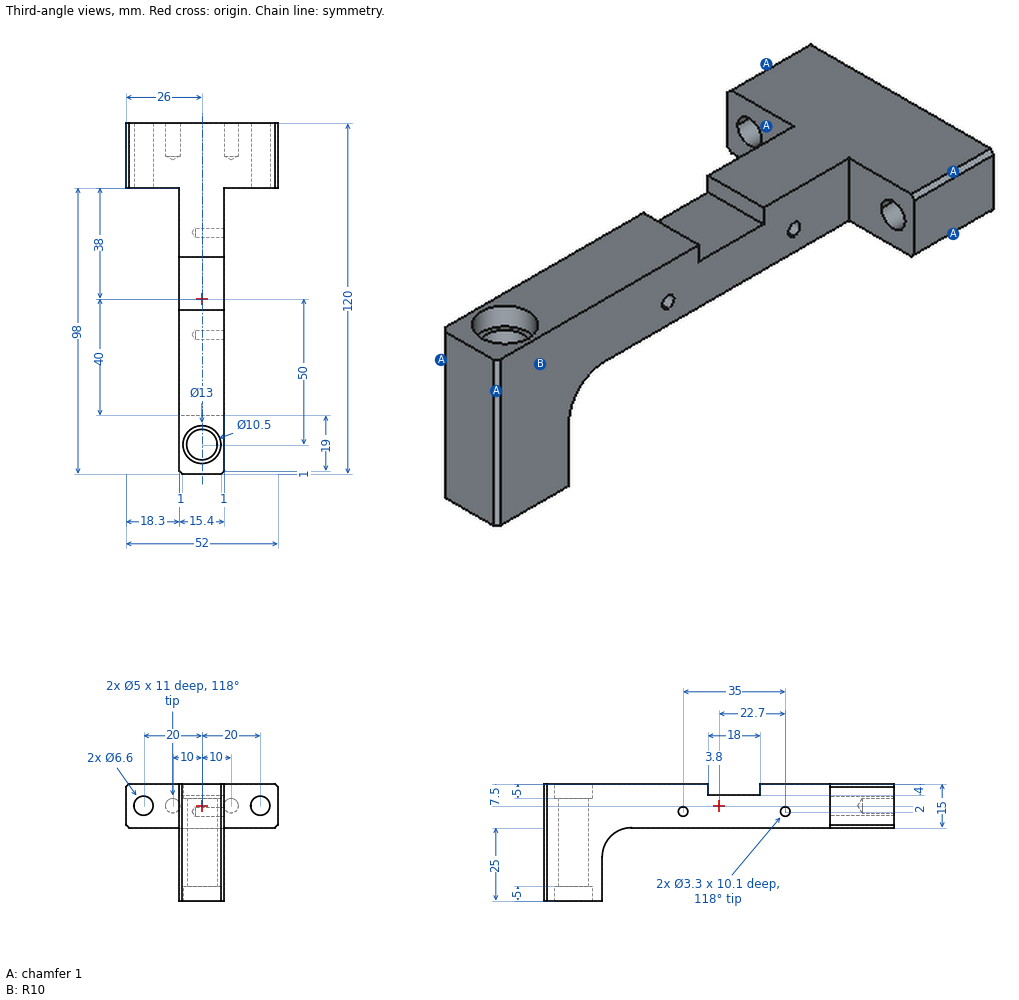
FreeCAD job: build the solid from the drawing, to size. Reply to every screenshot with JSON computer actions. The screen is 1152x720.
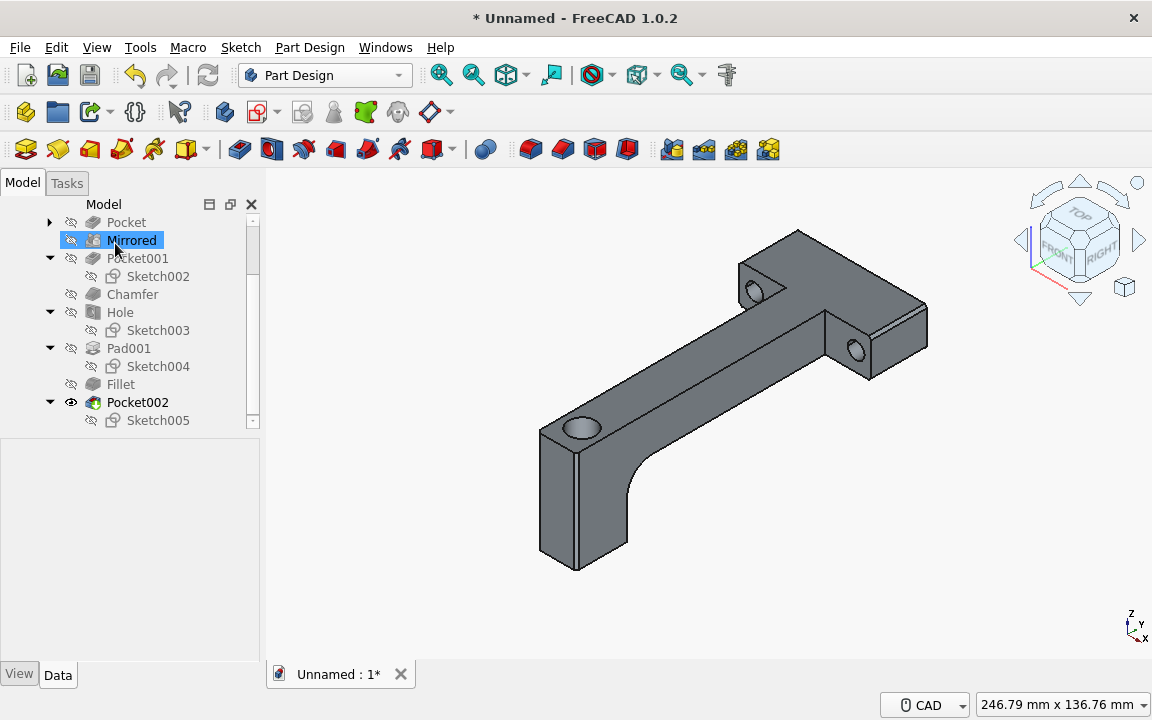
{"action": "left_click", "coordinate": [876, 299]}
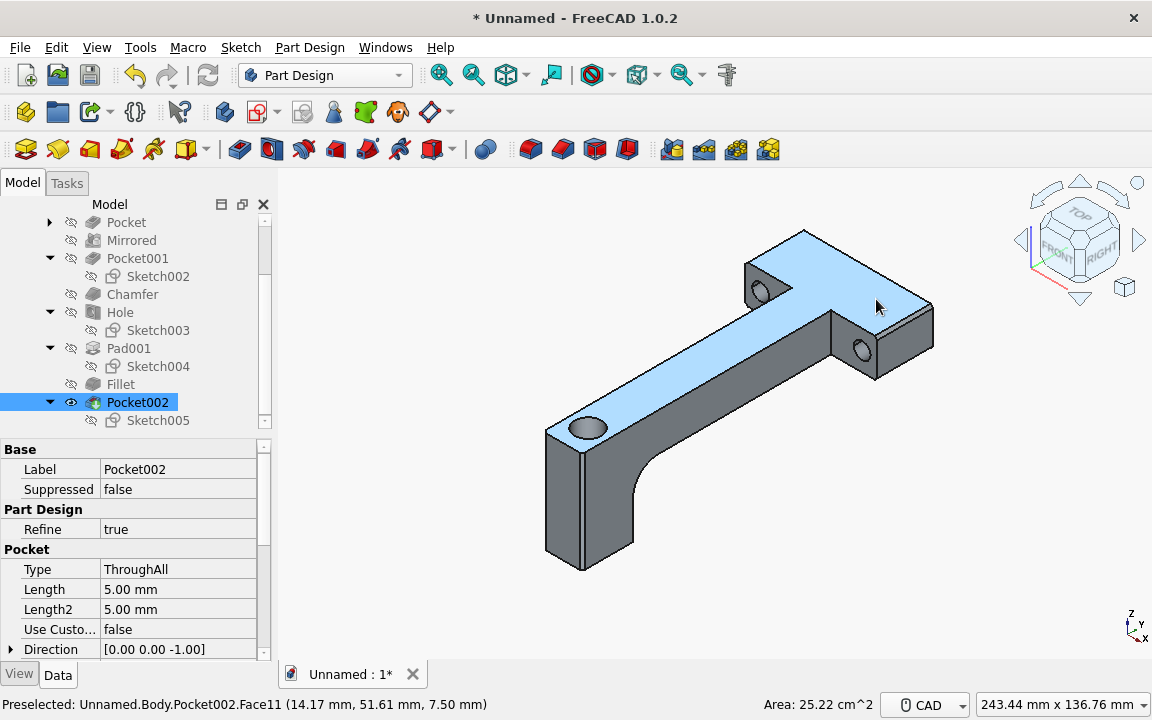
{"action": "left_click", "coordinate": [258, 112]}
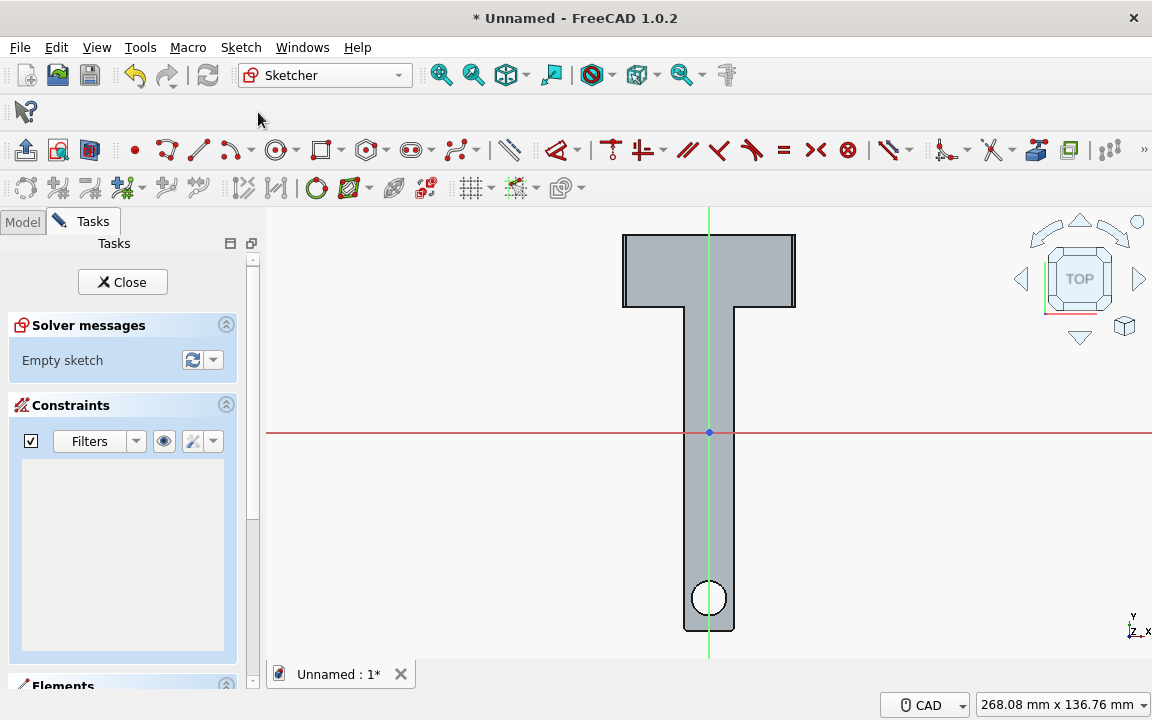
{"action": "scroll", "coordinate": [723, 631], "scroll_direction": "up", "scroll_amount": 9}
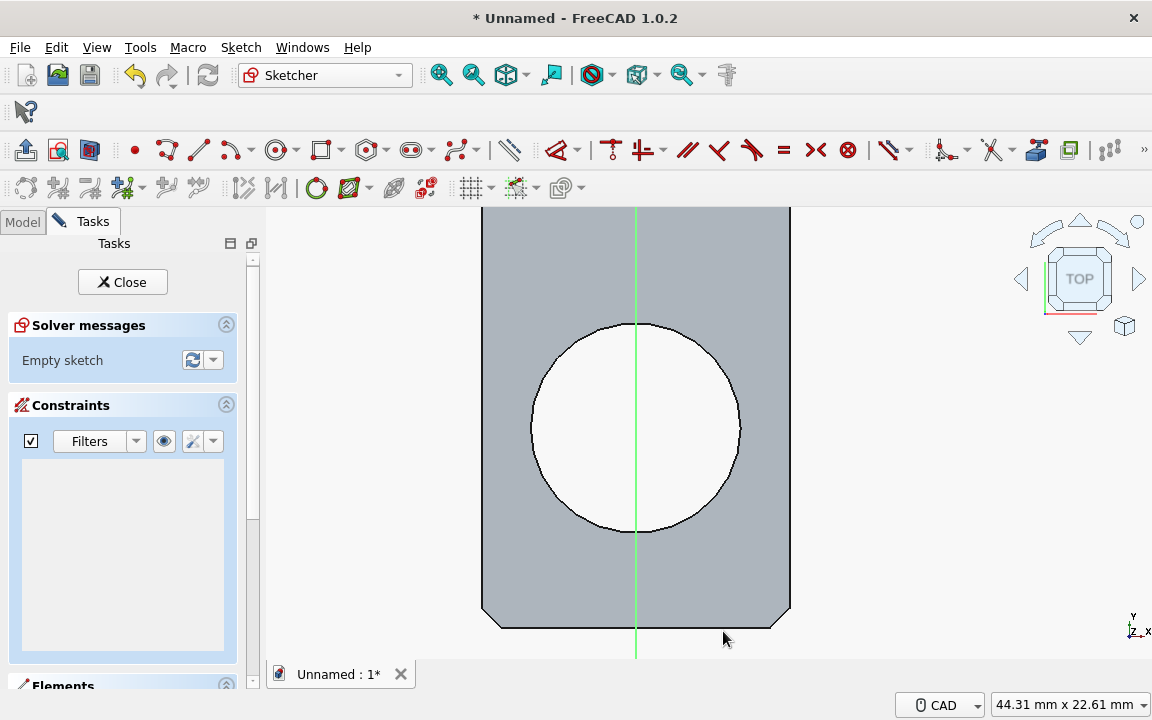
{"action": "left_click", "coordinate": [276, 150]}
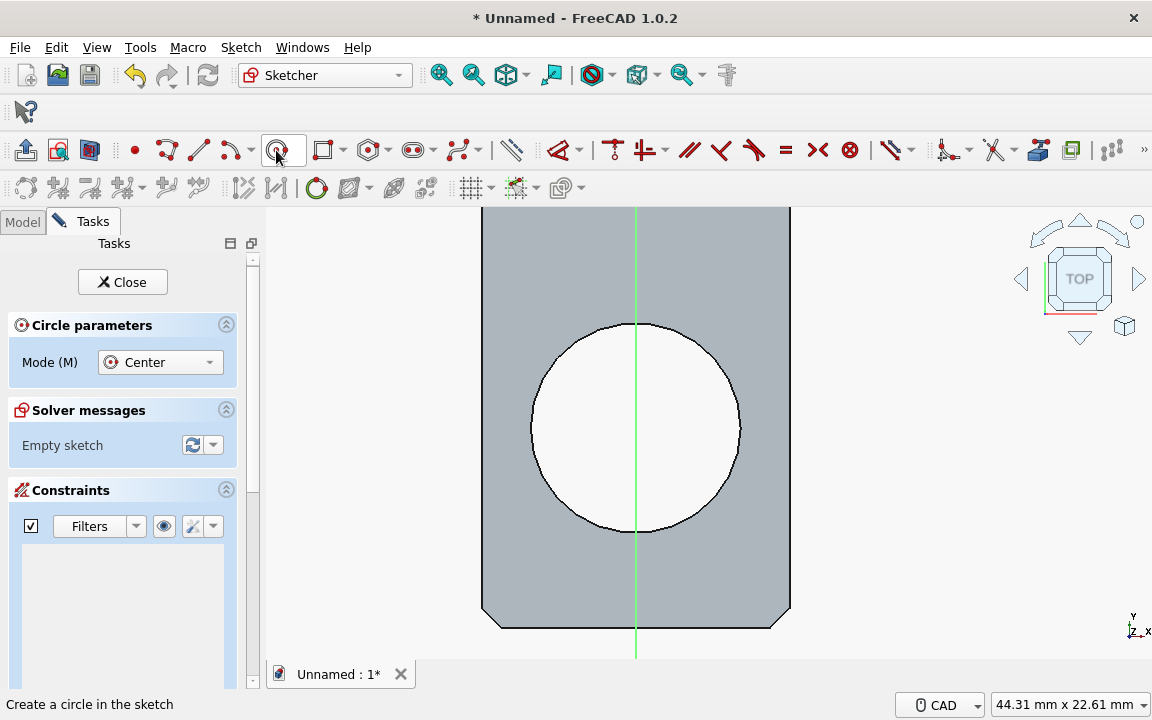
{"action": "left_click", "coordinate": [636, 428]}
{"action": "mouse_move", "coordinate": [728, 336]}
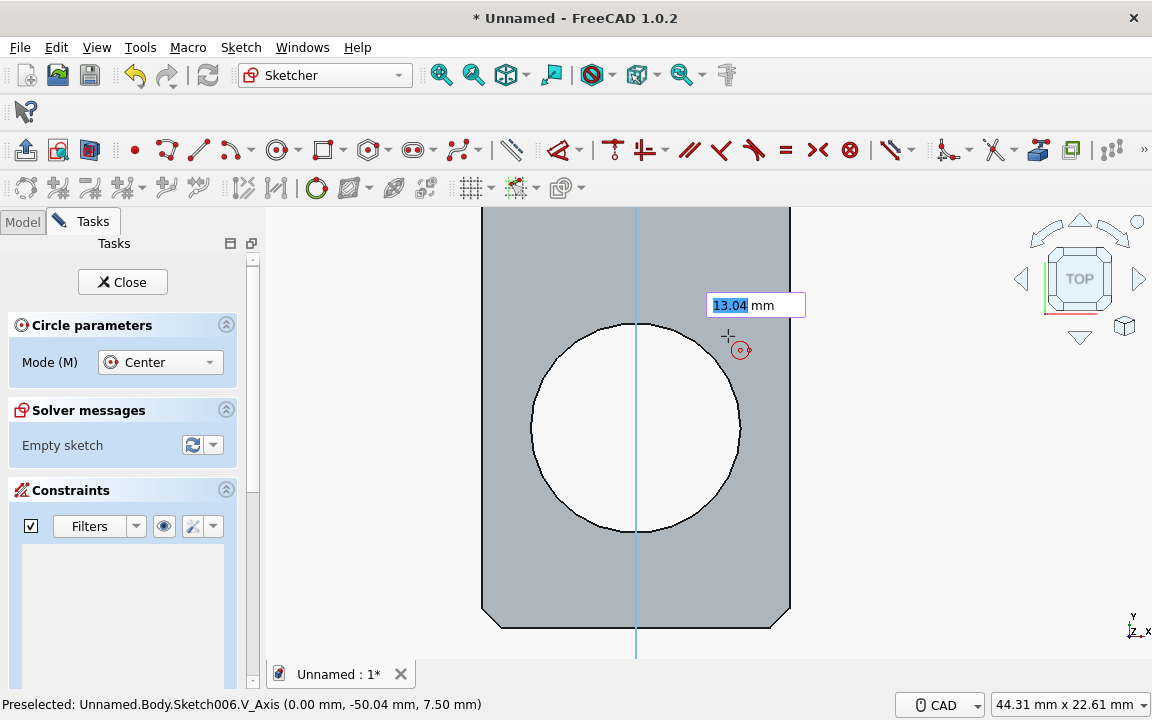
{"action": "type", "text": "13"}
{"action": "key", "text": "Return"}
{"action": "key", "text": "Escape"}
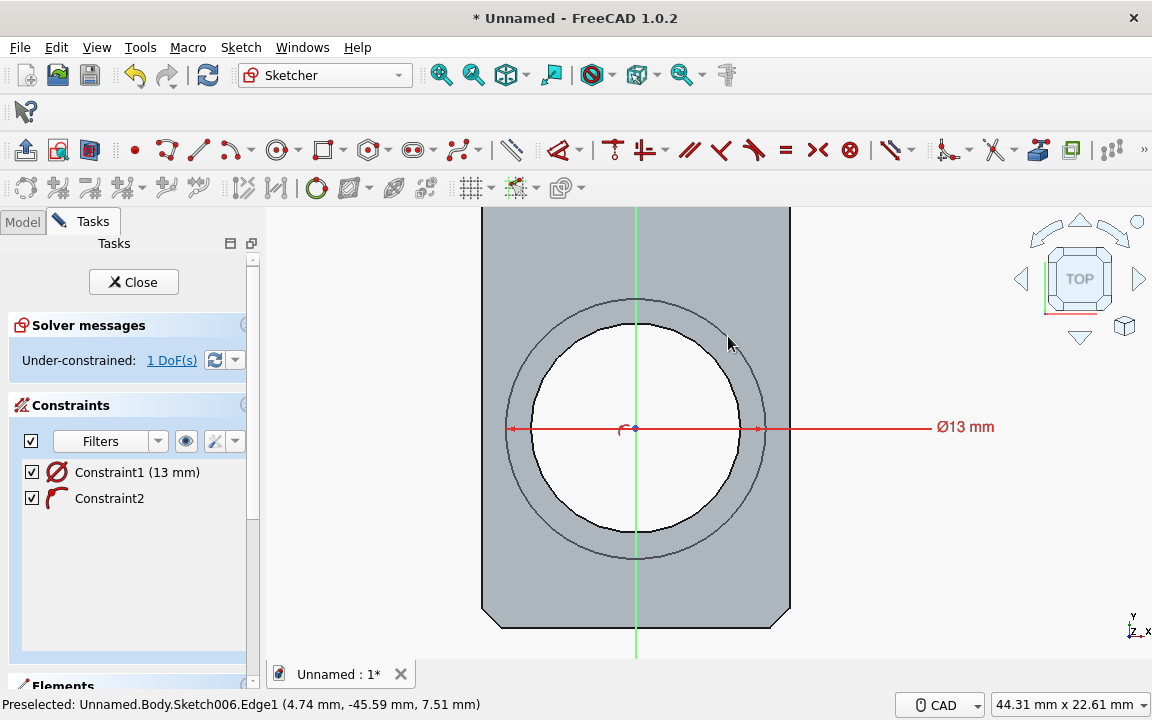
{"action": "left_click", "coordinate": [558, 150]}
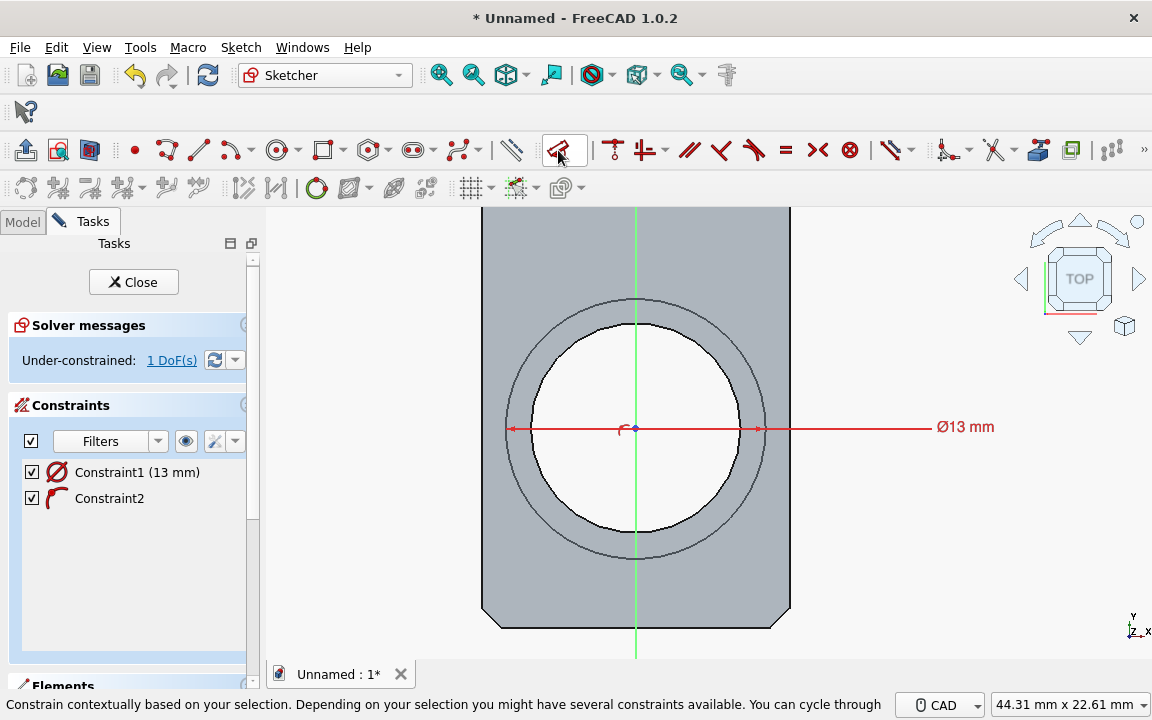
{"action": "left_click", "coordinate": [636, 429]}
{"action": "left_click", "coordinate": [670, 332]}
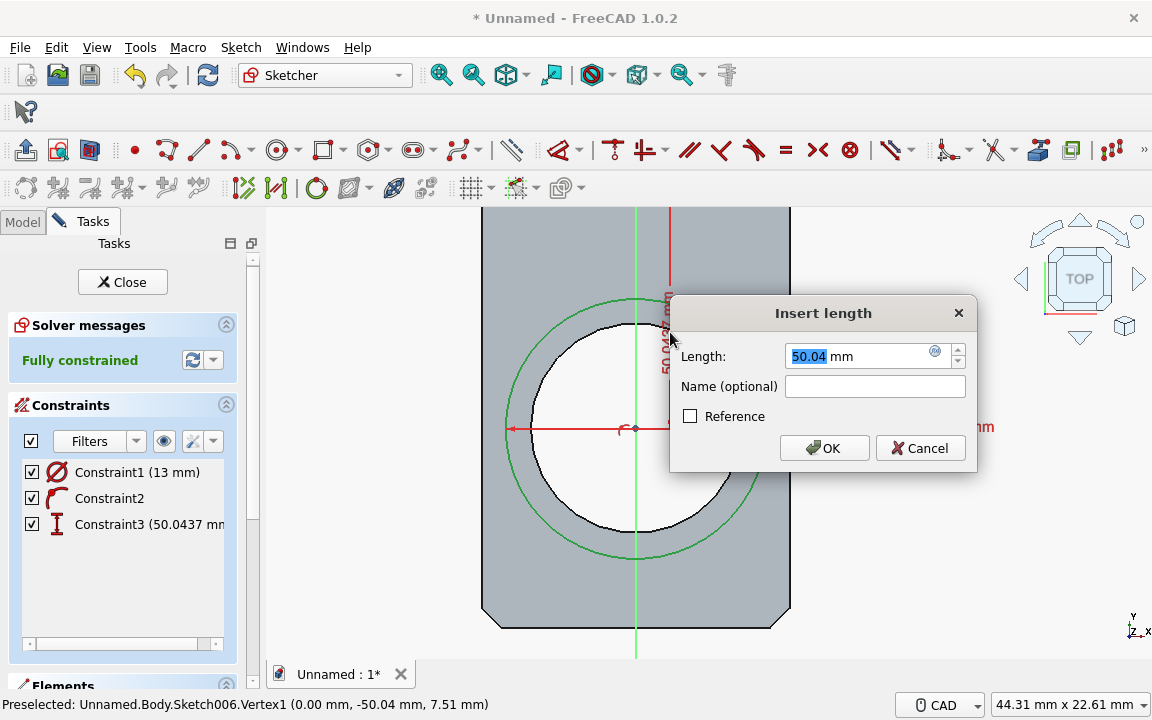
{"action": "type", "text": "50"}
{"action": "key", "text": "Return"}
{"action": "key", "text": "Escape"}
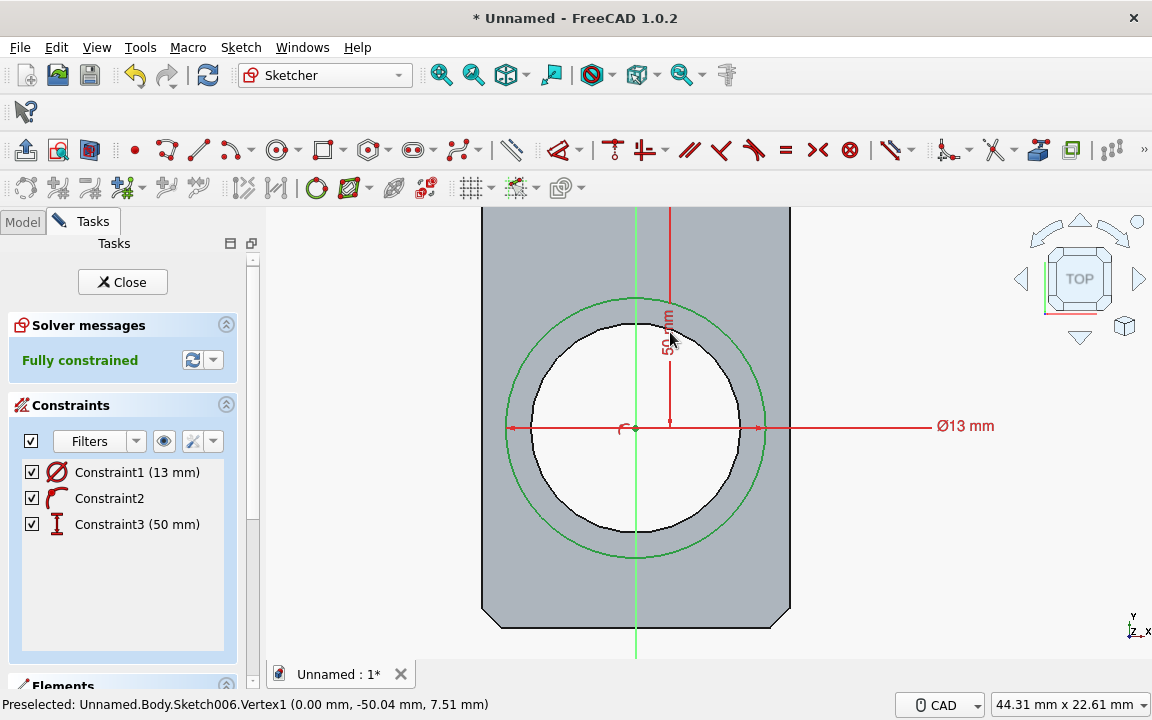
{"action": "left_click", "coordinate": [123, 282]}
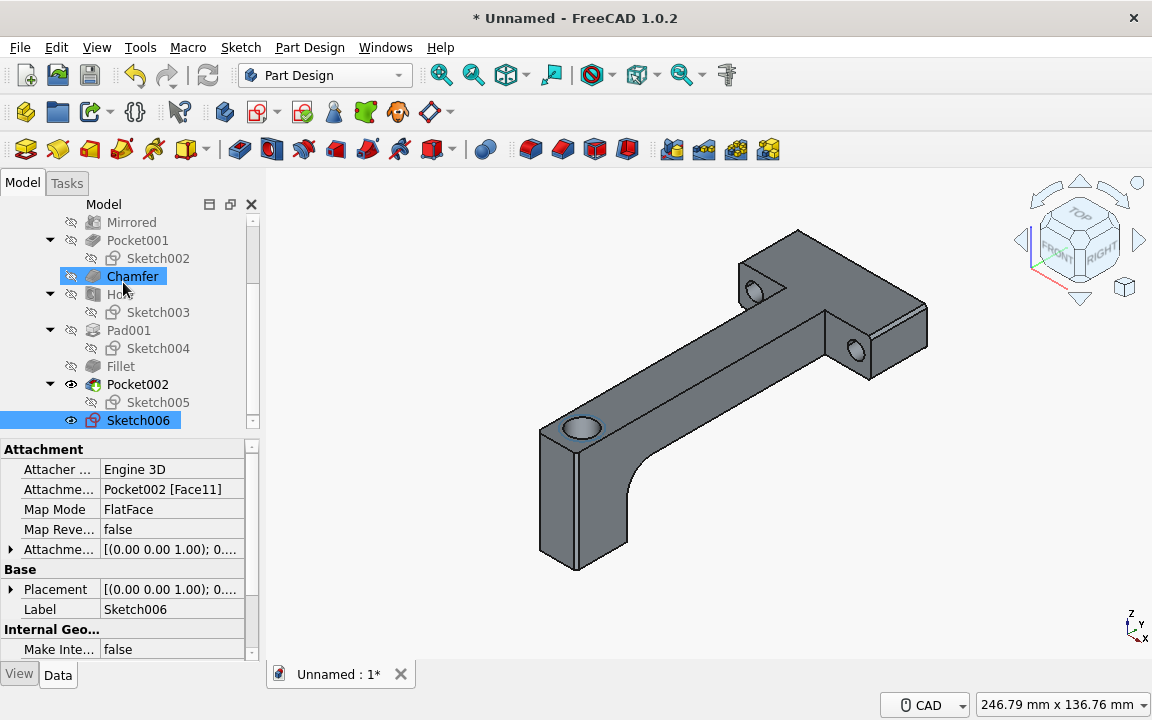
{"action": "left_click", "coordinate": [240, 150]}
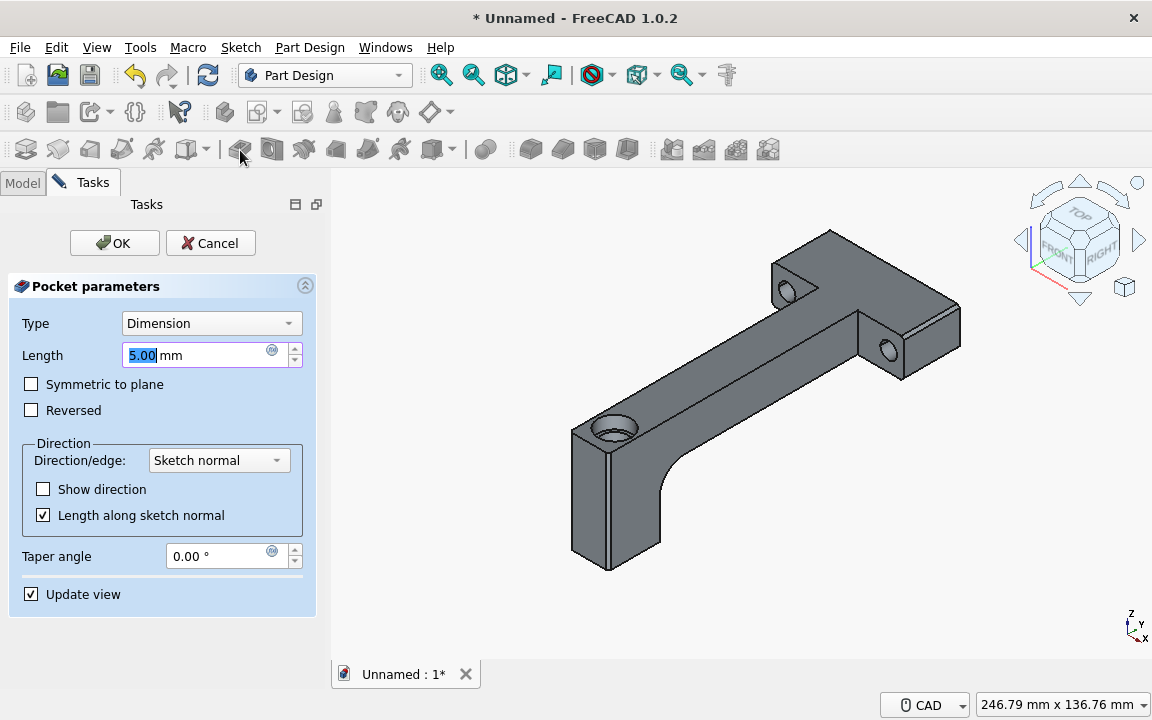
{"action": "type", "text": "5"}
{"action": "key", "text": "Tab"}